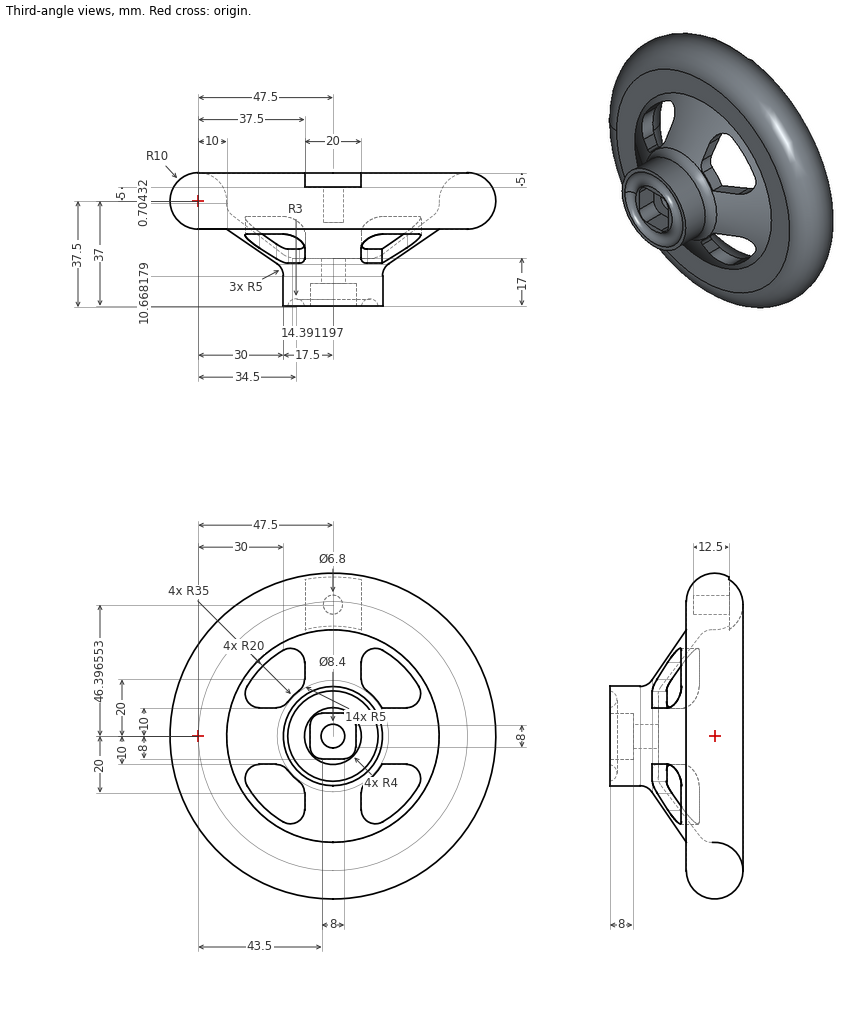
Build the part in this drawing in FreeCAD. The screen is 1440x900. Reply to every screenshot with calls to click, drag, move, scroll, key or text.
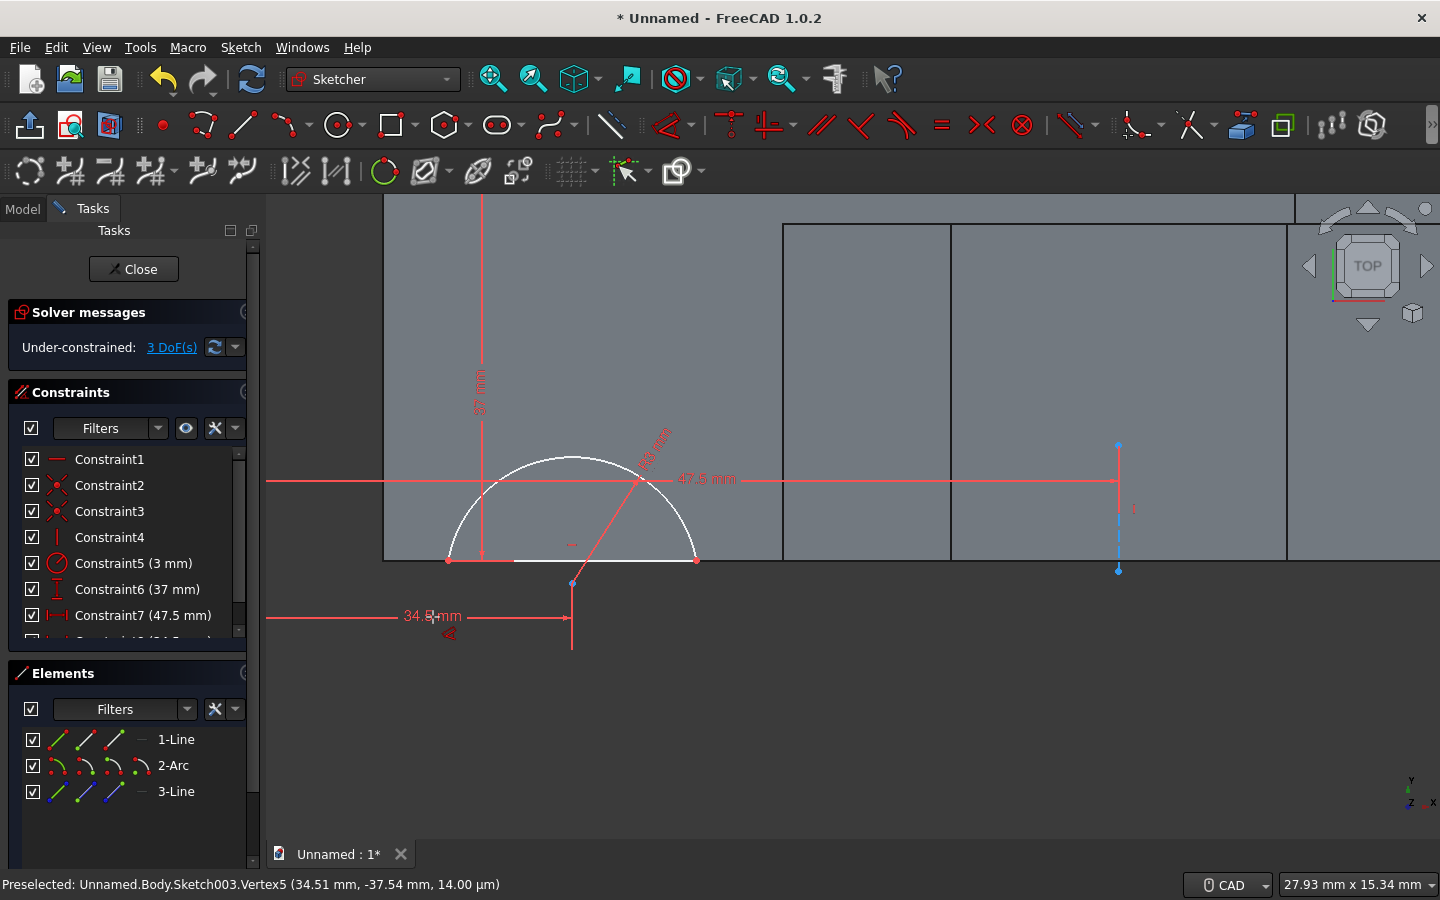
click(572, 583)
click(606, 403)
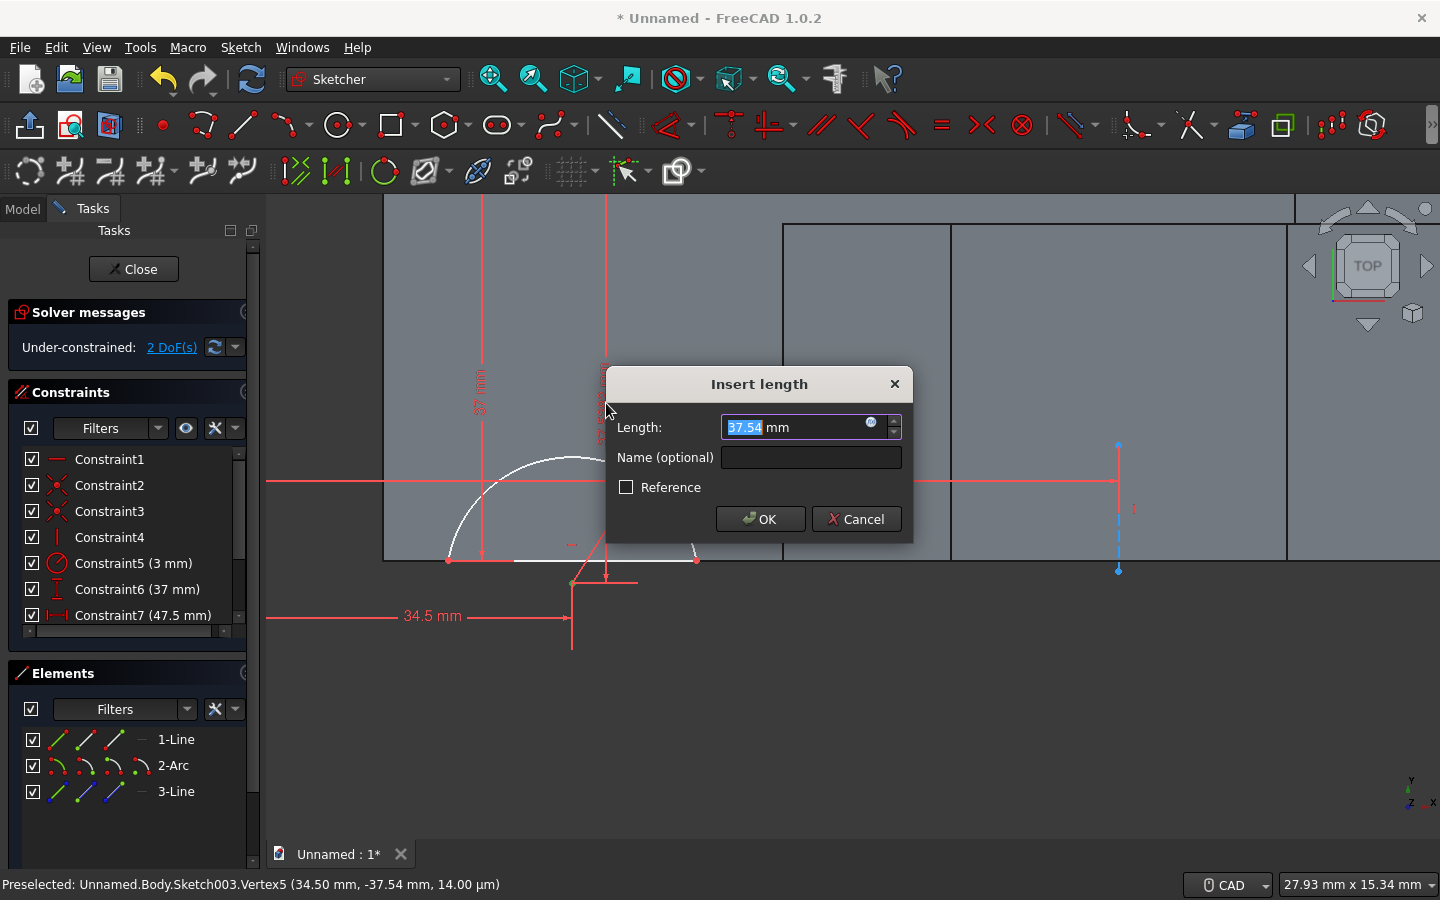
text(37.5)
key(Return)
key(Escape)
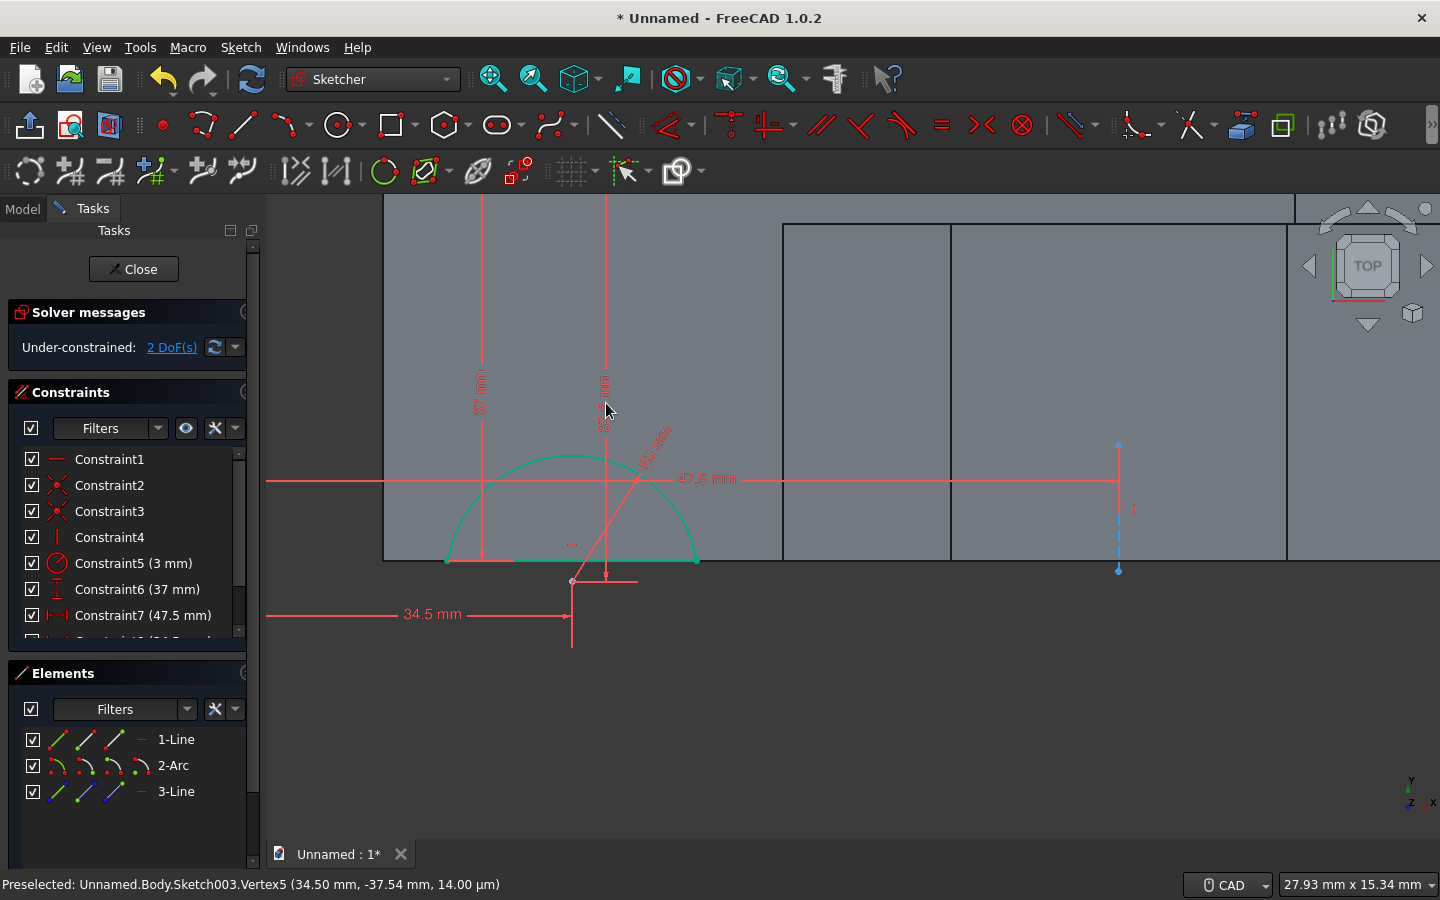
click(134, 269)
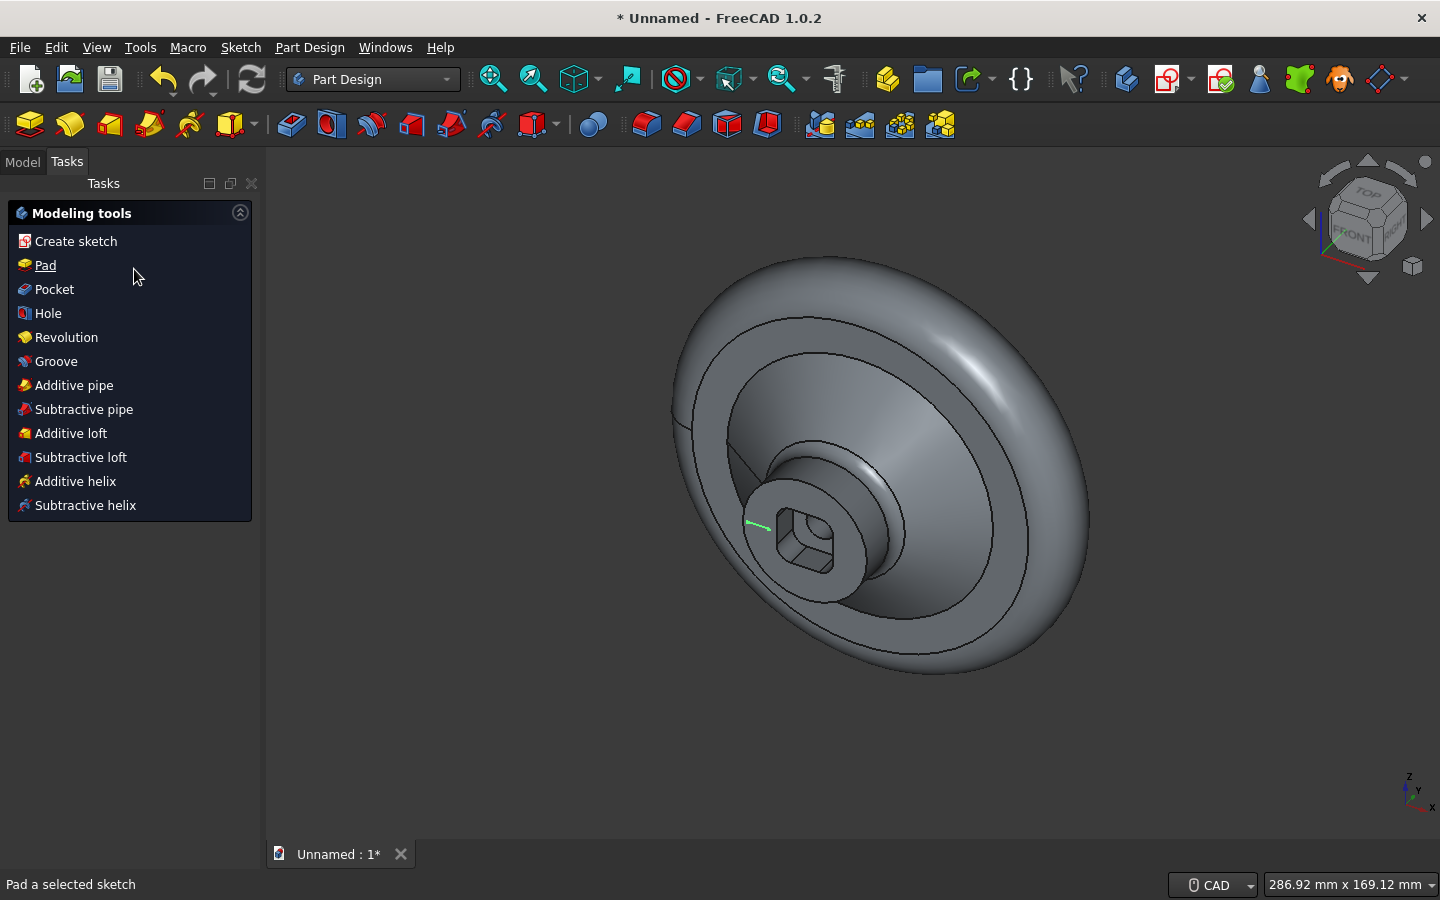
click(372, 124)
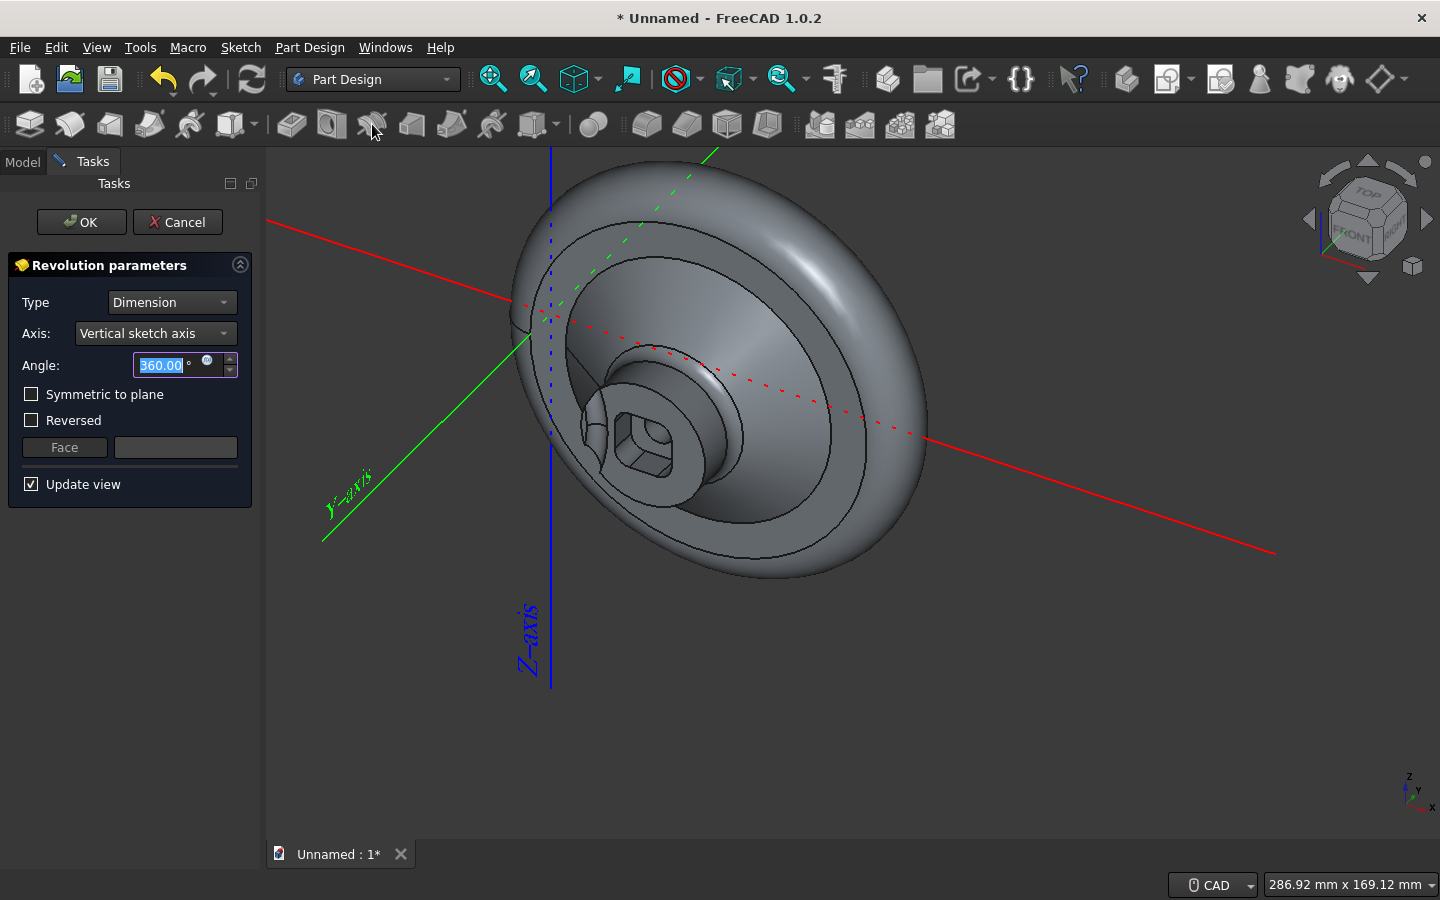
click(156, 334)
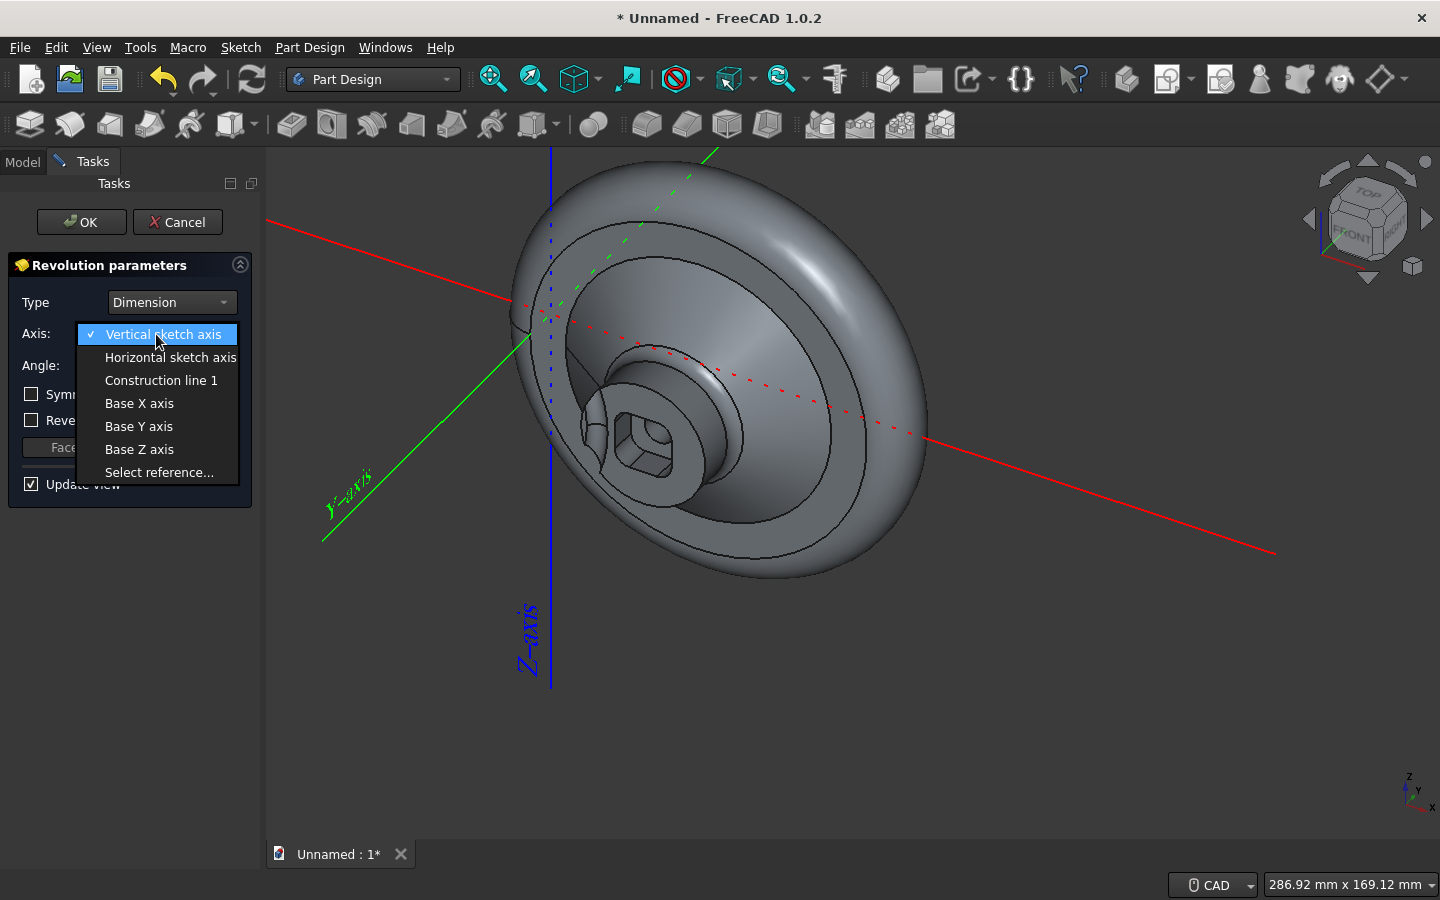
click(156, 380)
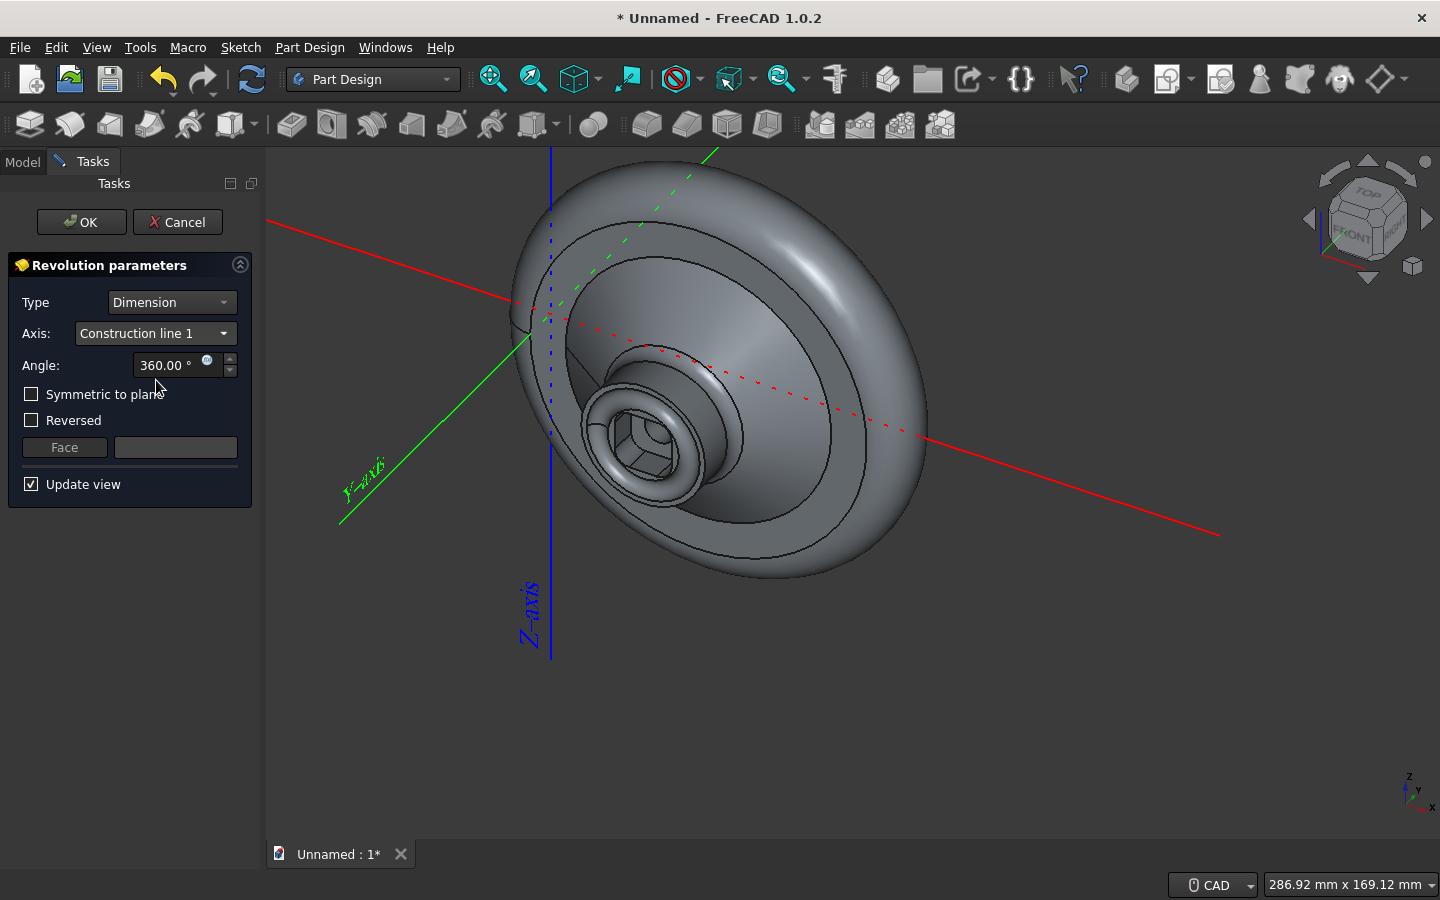
click(82, 222)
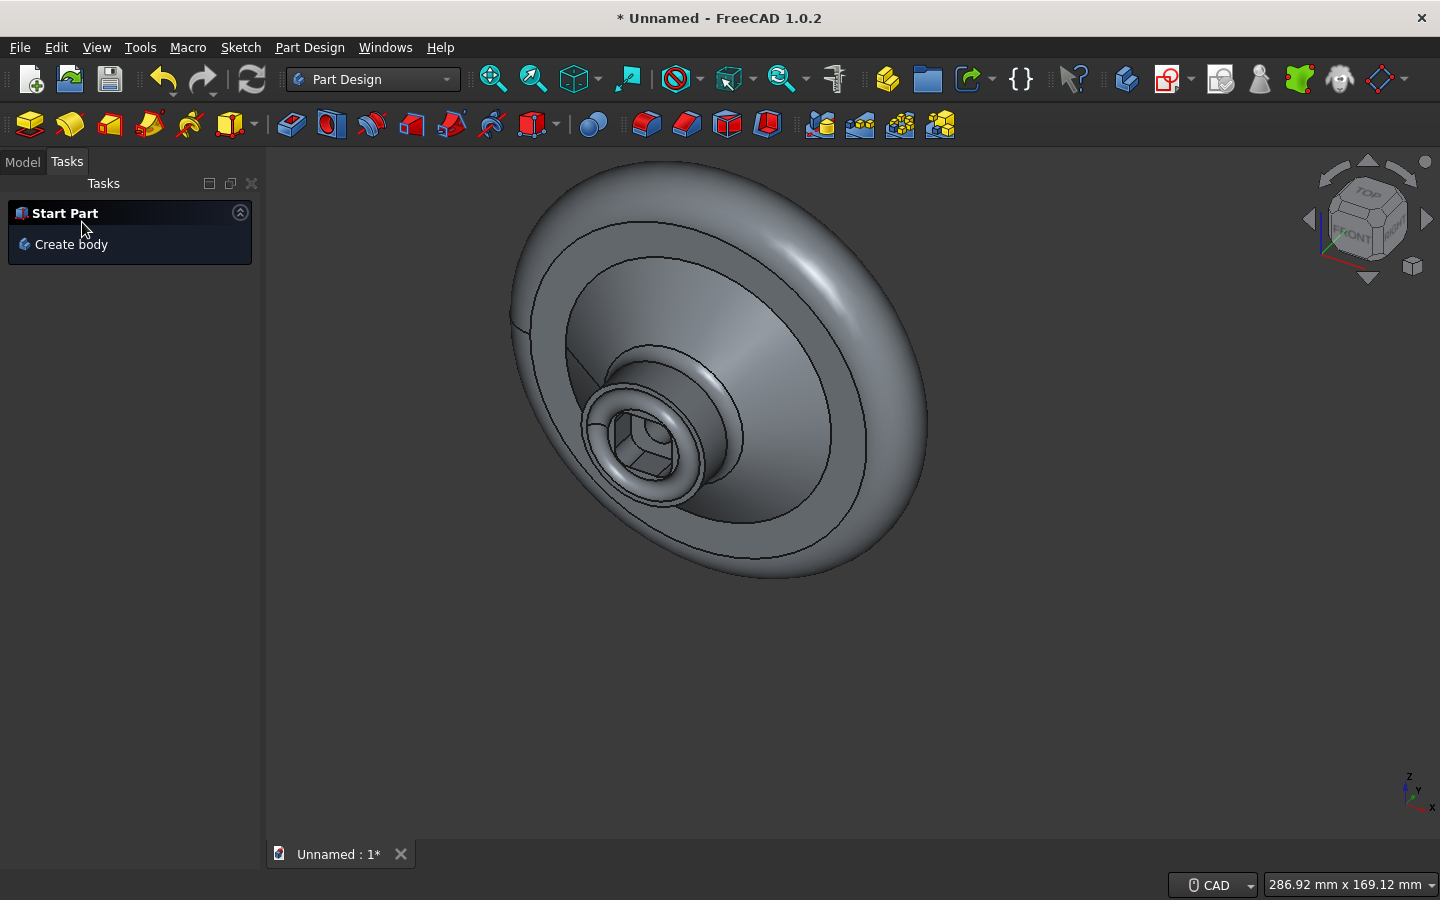
click(494, 80)